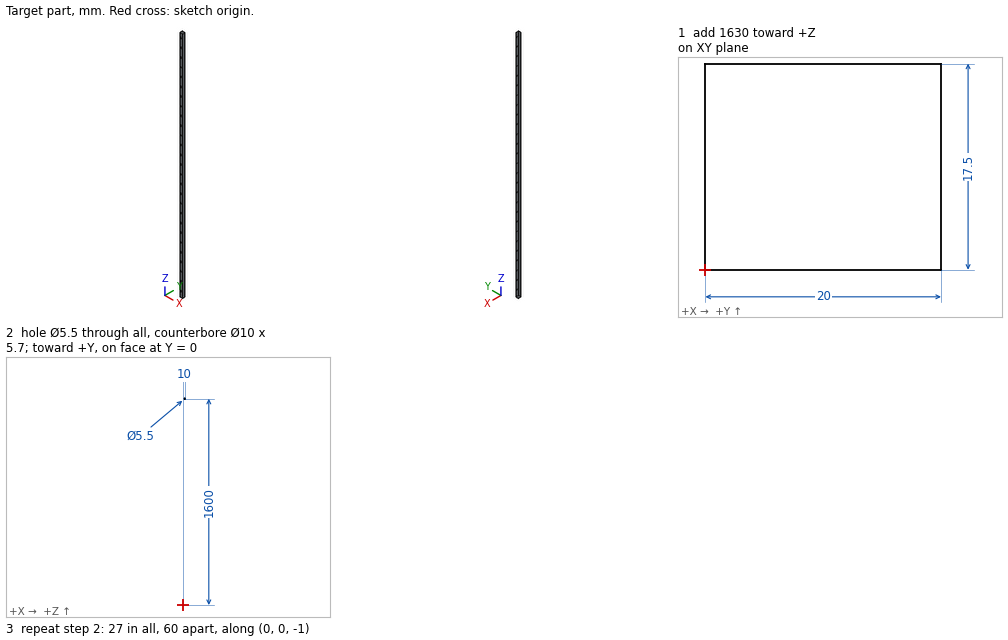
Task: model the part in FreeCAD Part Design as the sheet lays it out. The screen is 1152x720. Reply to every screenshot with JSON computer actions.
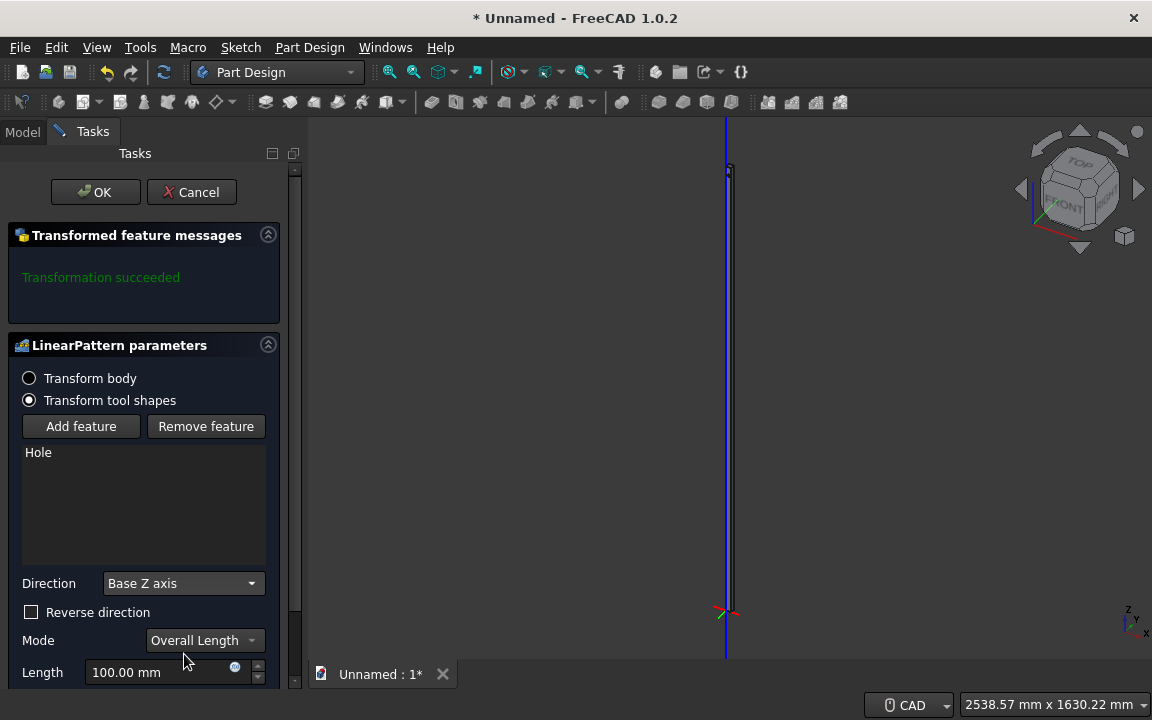
{"action": "left_click", "coordinate": [206, 640]}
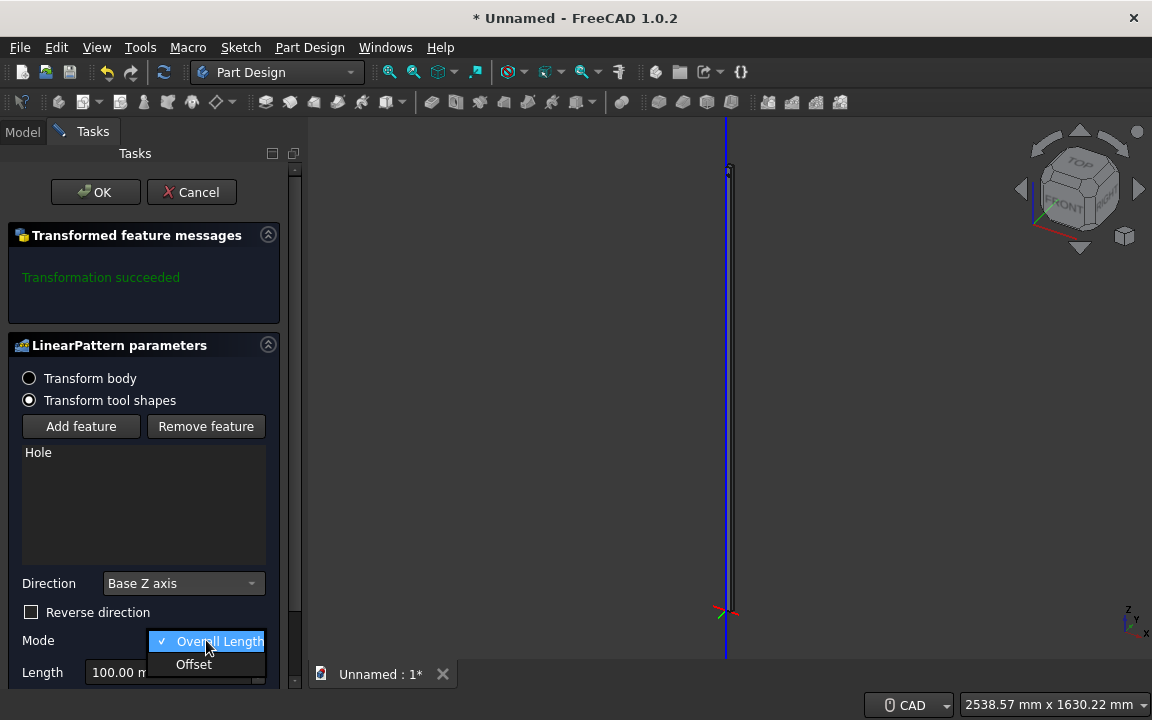
{"action": "left_click", "coordinate": [206, 664]}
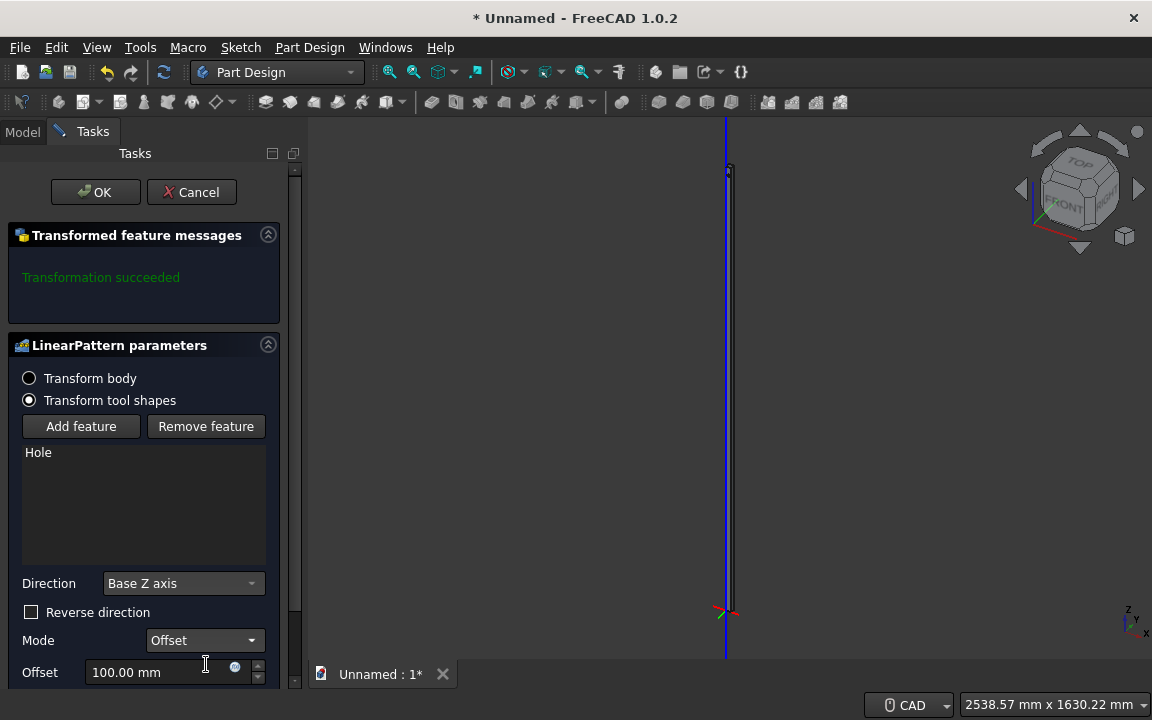
{"action": "triple_click", "coordinate": [168, 672]}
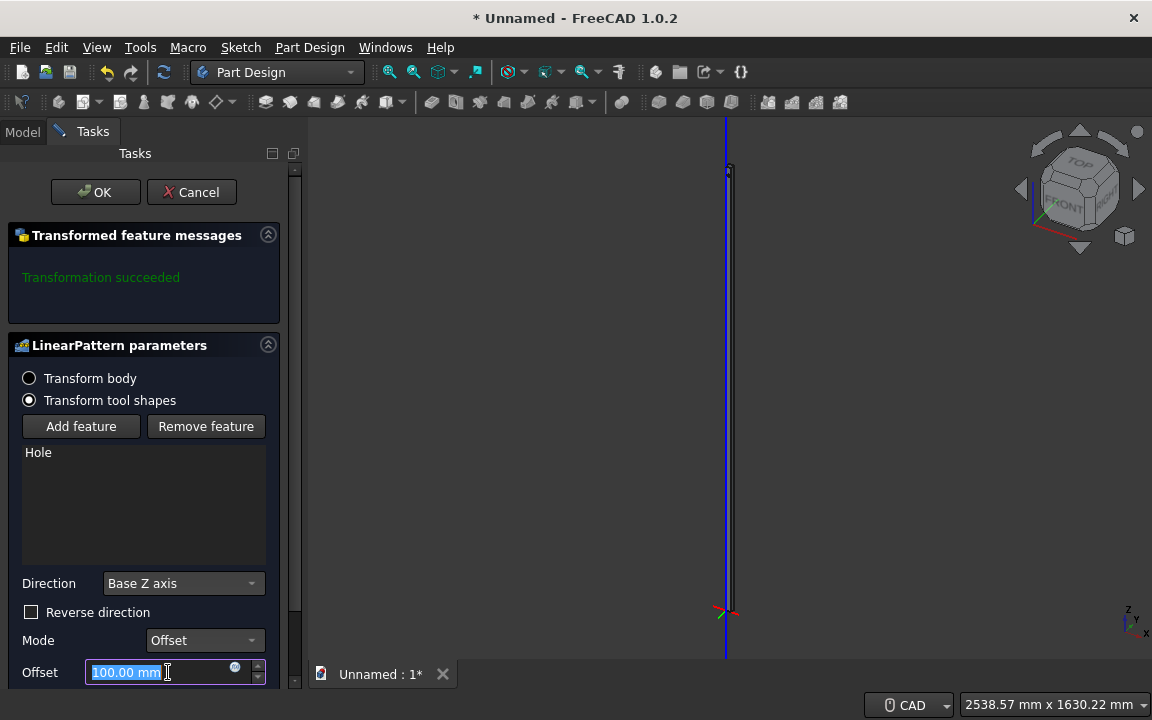
{"action": "type", "text": "60"}
{"action": "key", "text": "Tab"}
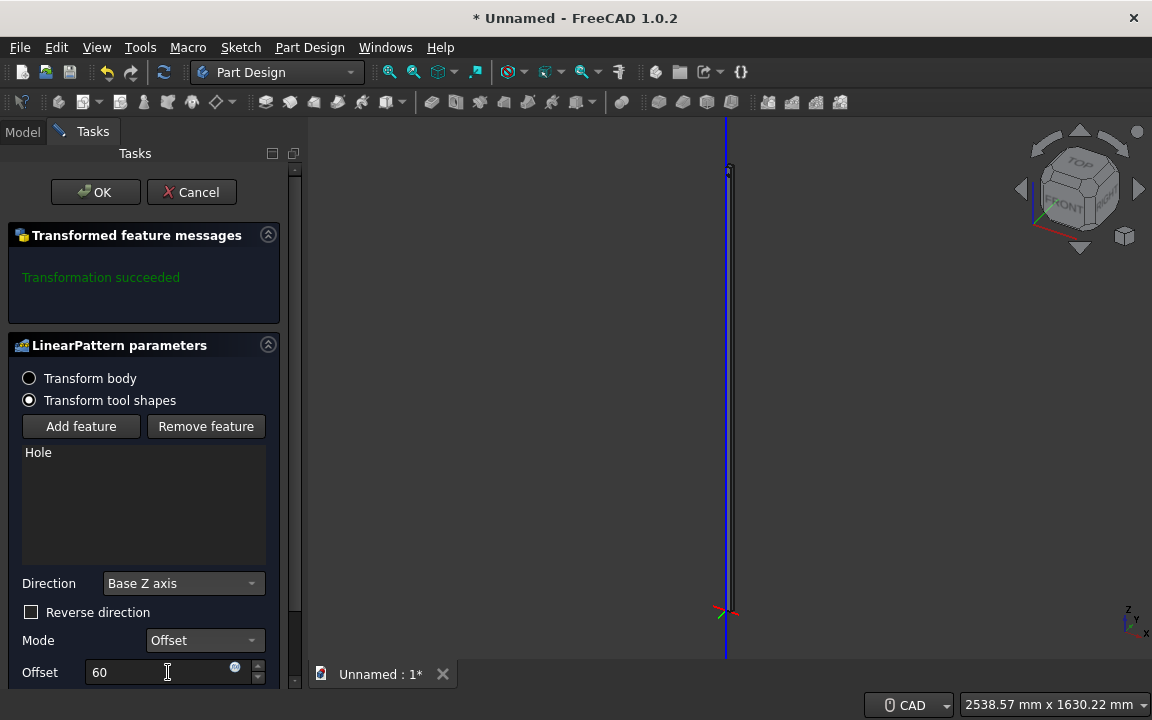
{"action": "scroll", "coordinate": [295, 426], "scroll_direction": "down", "scroll_amount": 2}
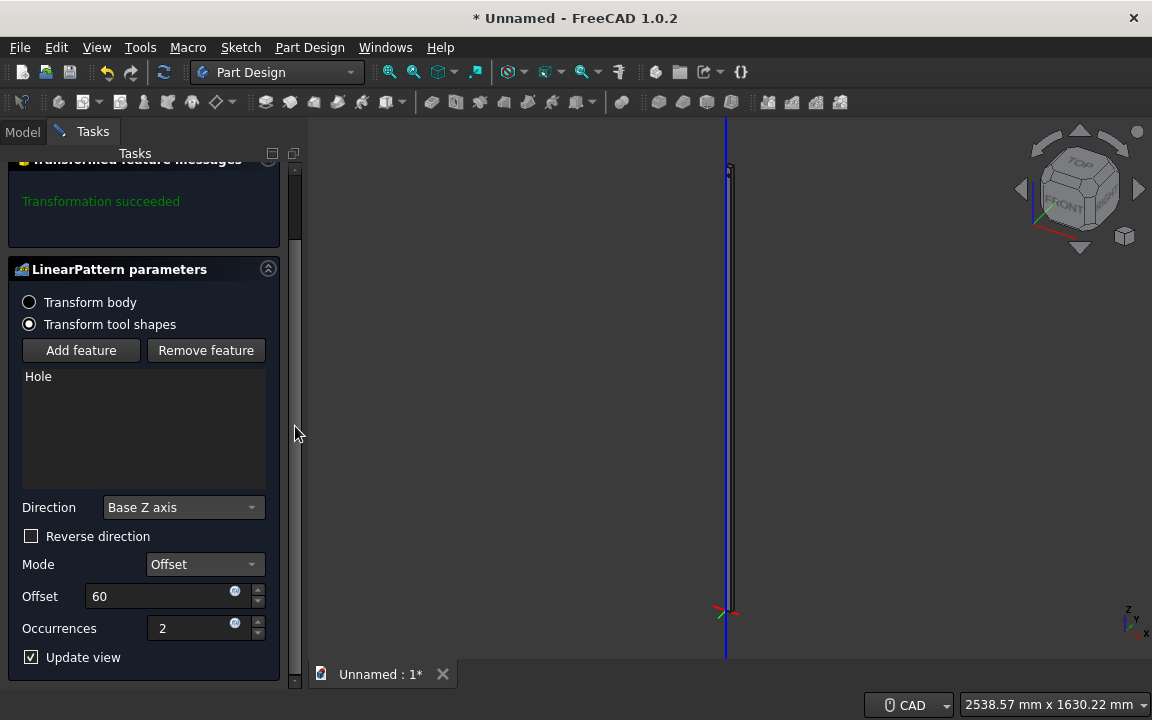
{"action": "triple_click", "coordinate": [198, 628]}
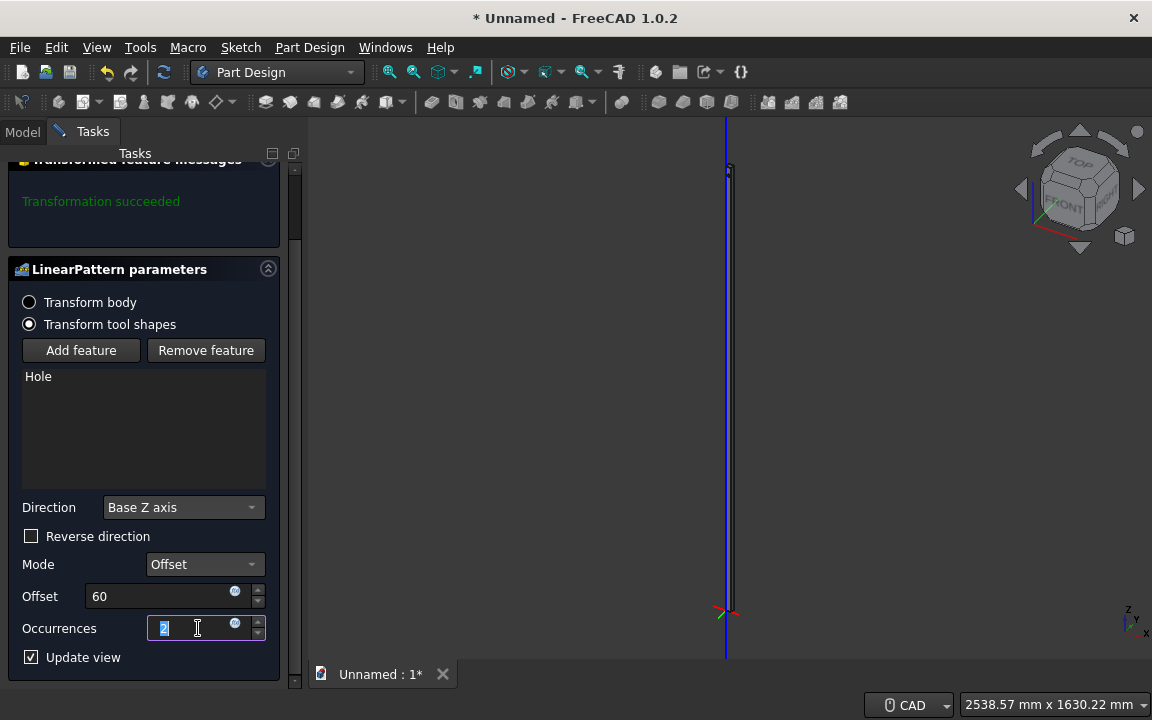
{"action": "type", "text": "27"}
{"action": "key", "text": "Tab"}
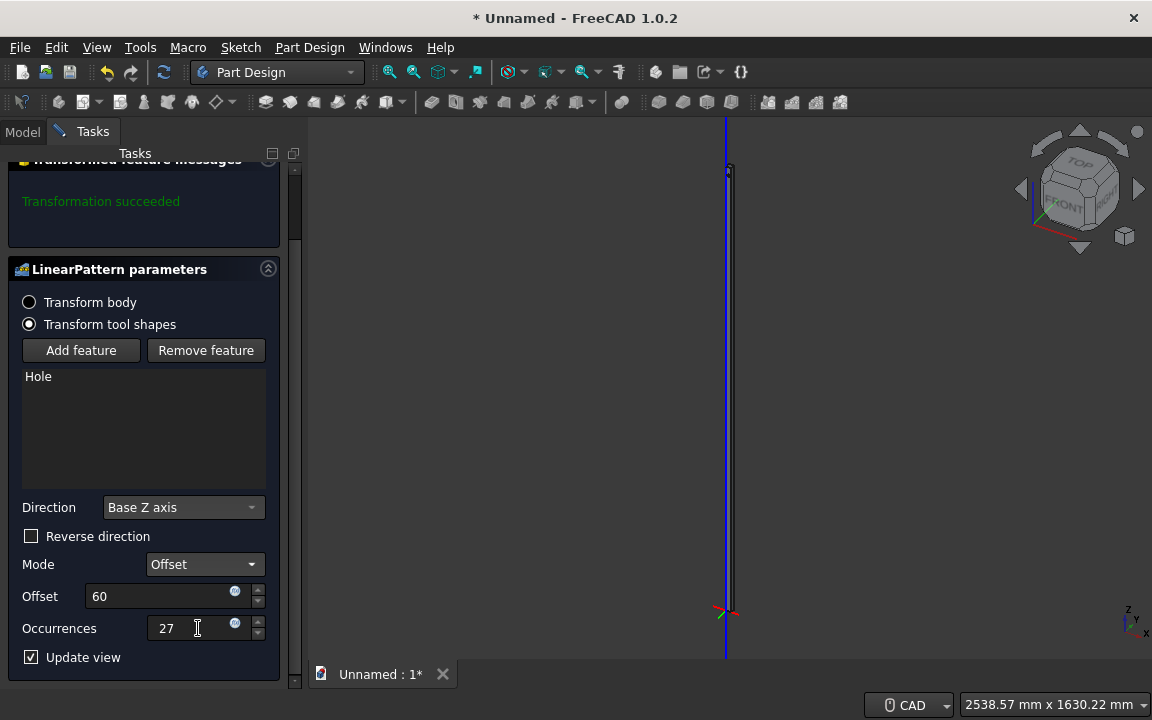
{"action": "left_click", "coordinate": [30, 536]}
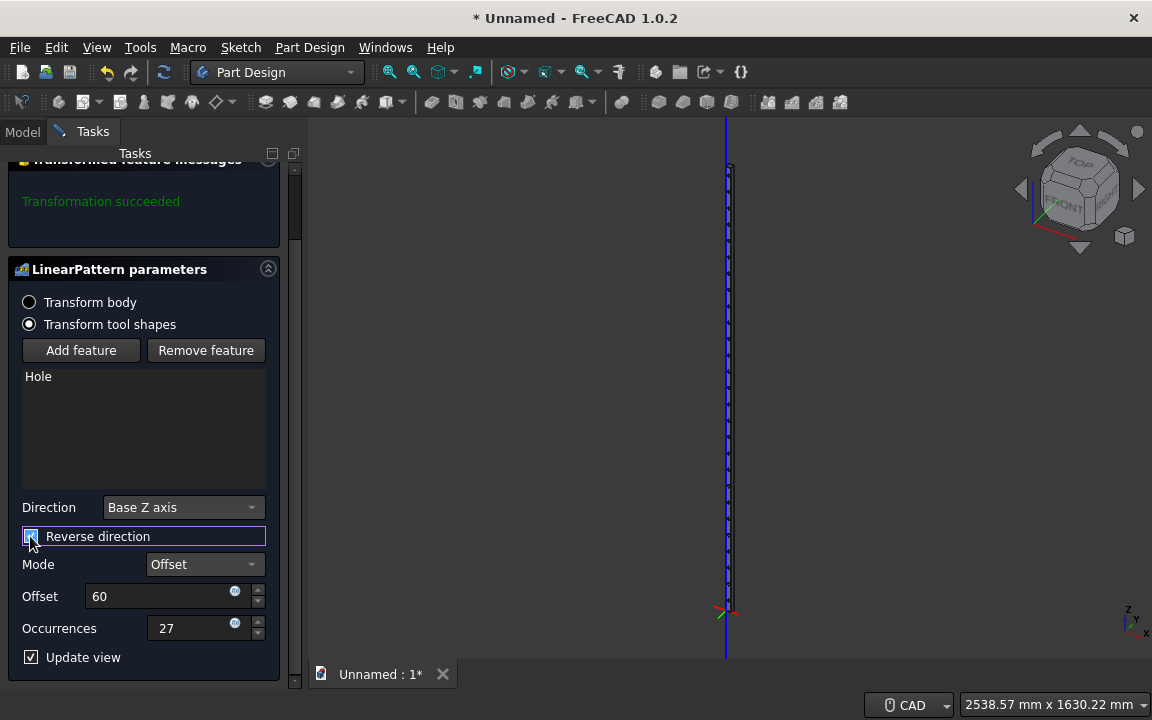
{"action": "scroll", "coordinate": [295, 426], "scroll_direction": "up", "scroll_amount": 3}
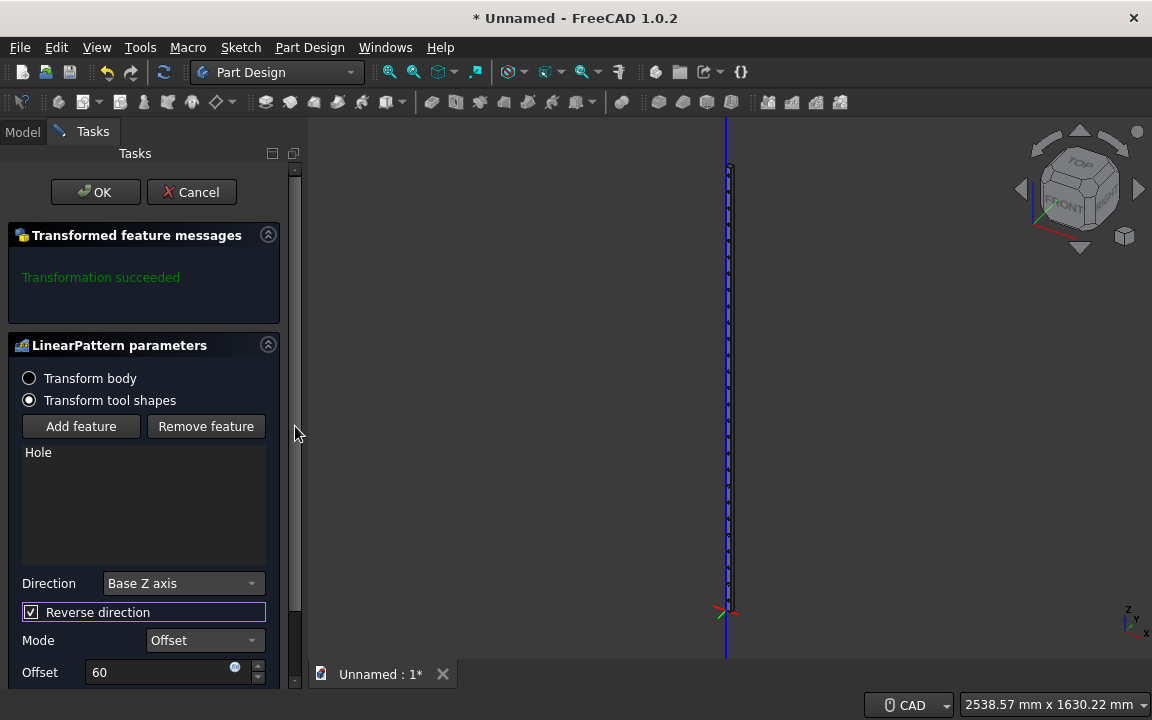
{"action": "left_click", "coordinate": [96, 192]}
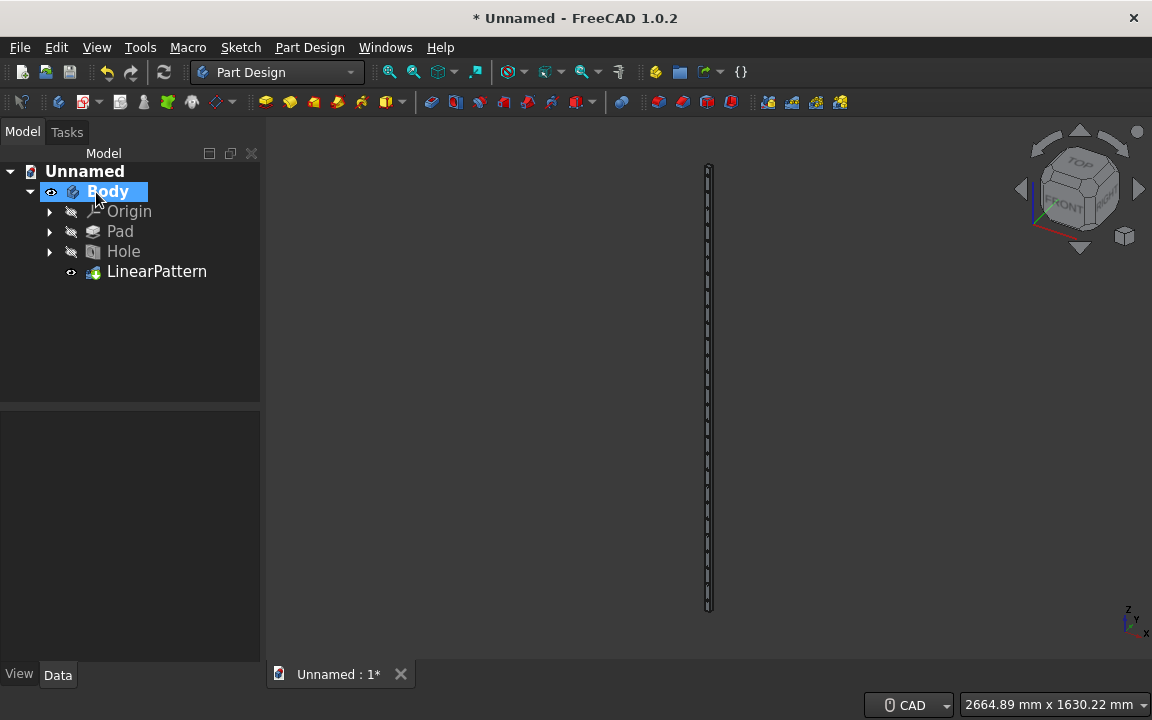
{"action": "key", "text": "0"}